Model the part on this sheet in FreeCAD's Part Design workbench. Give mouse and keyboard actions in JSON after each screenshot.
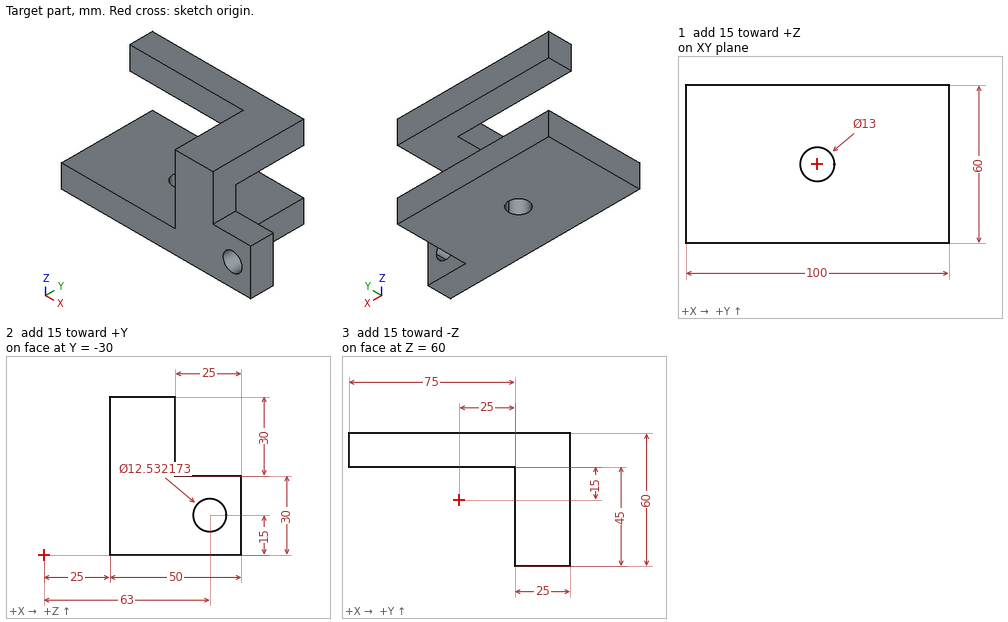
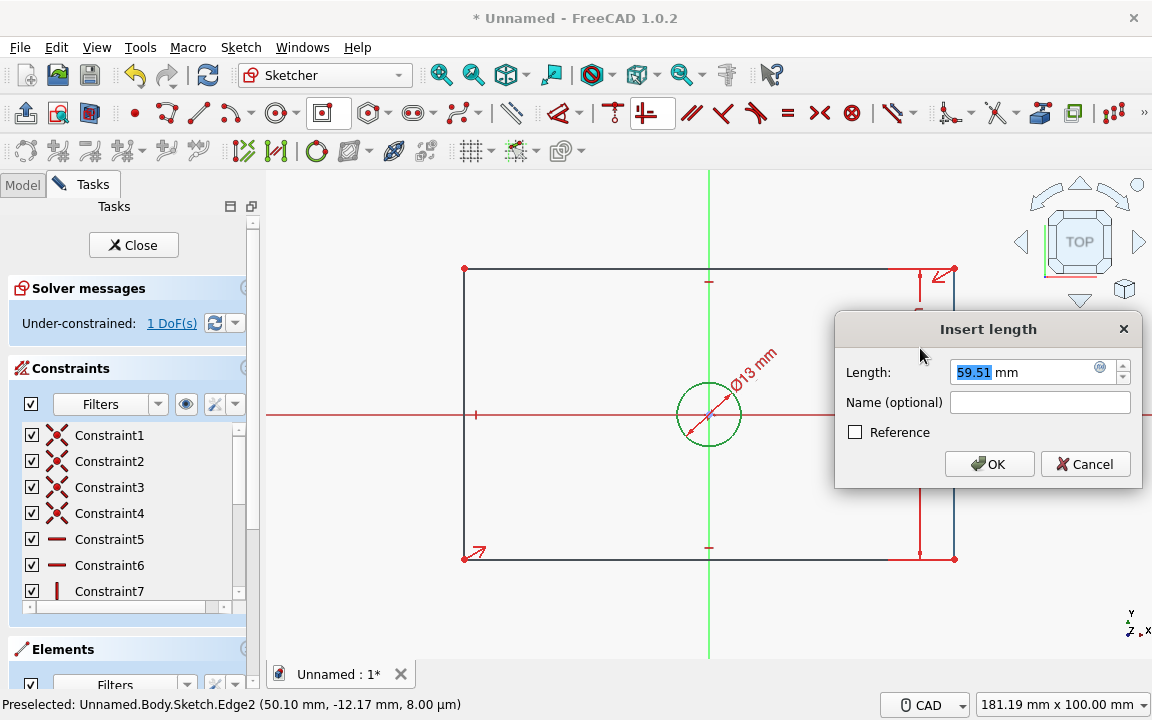
{"action": "type", "text": "60"}
{"action": "key", "text": "Return"}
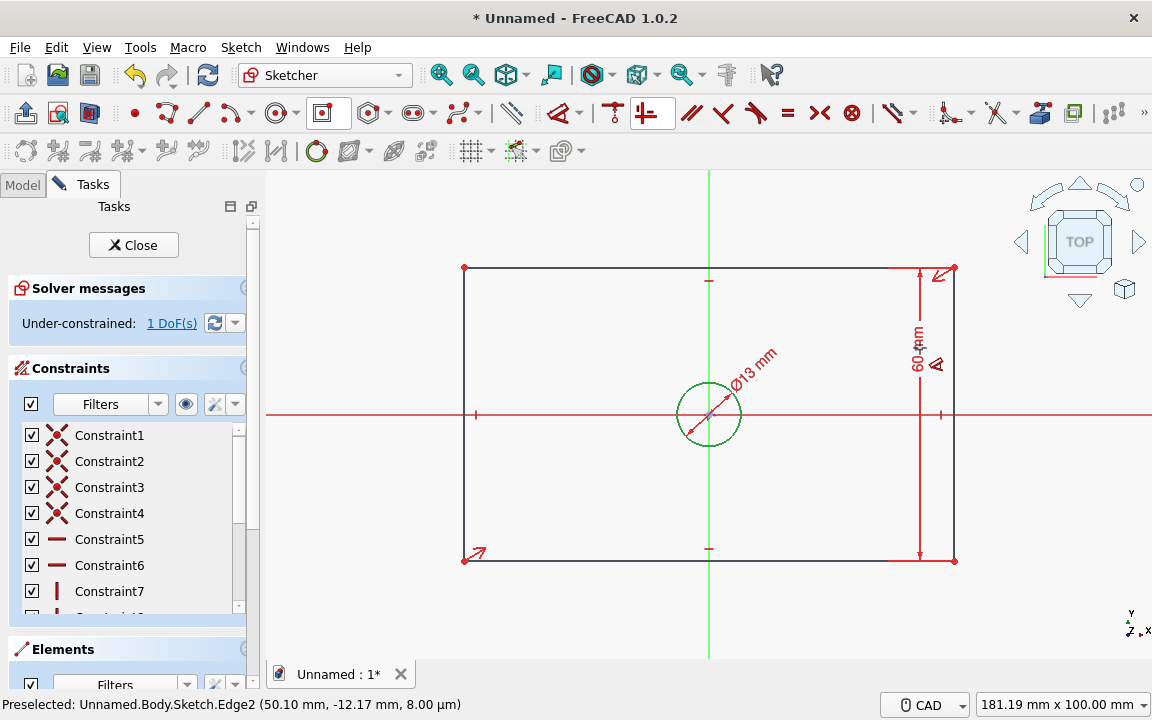
{"action": "left_click", "coordinate": [611, 561]}
{"action": "left_click", "coordinate": [596, 595]}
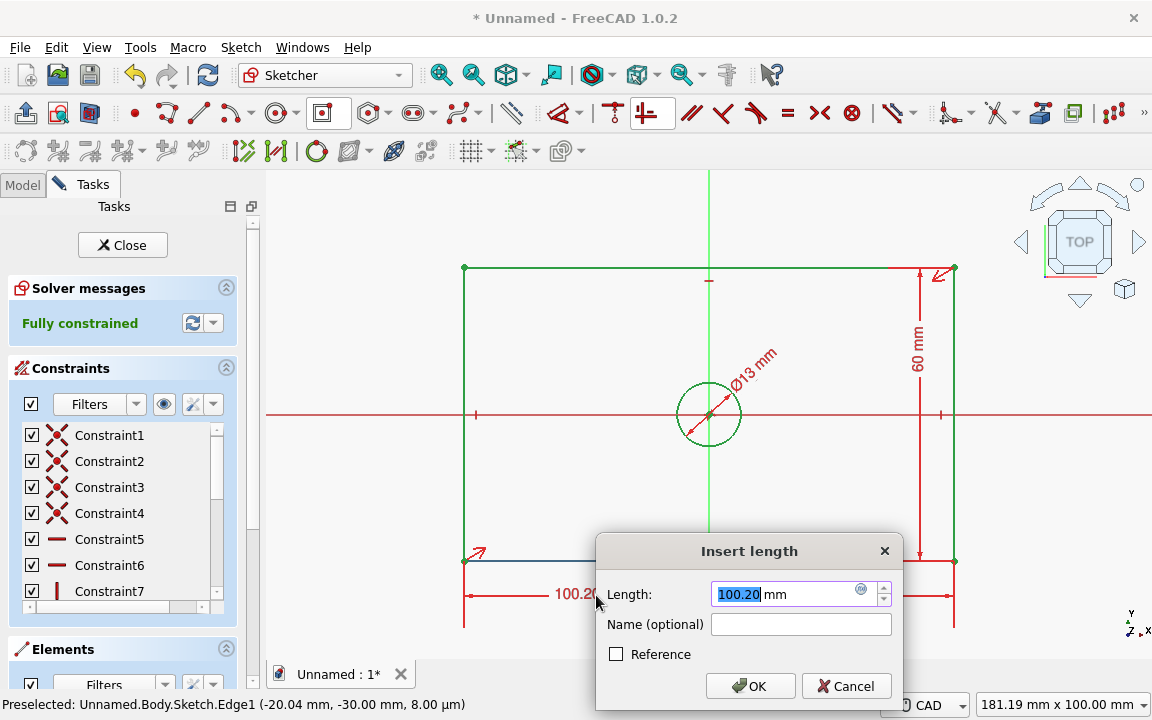
{"action": "type", "text": "100"}
{"action": "key", "text": "Return"}
{"action": "key", "text": "Escape"}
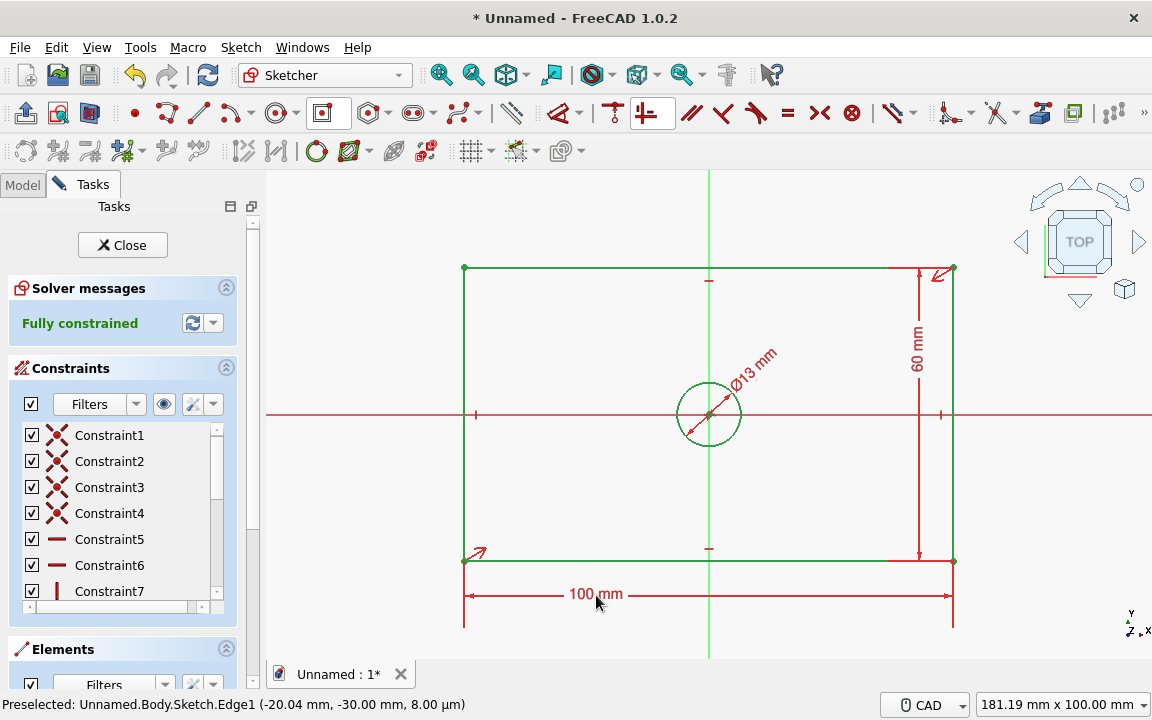
{"action": "left_click", "coordinate": [123, 245]}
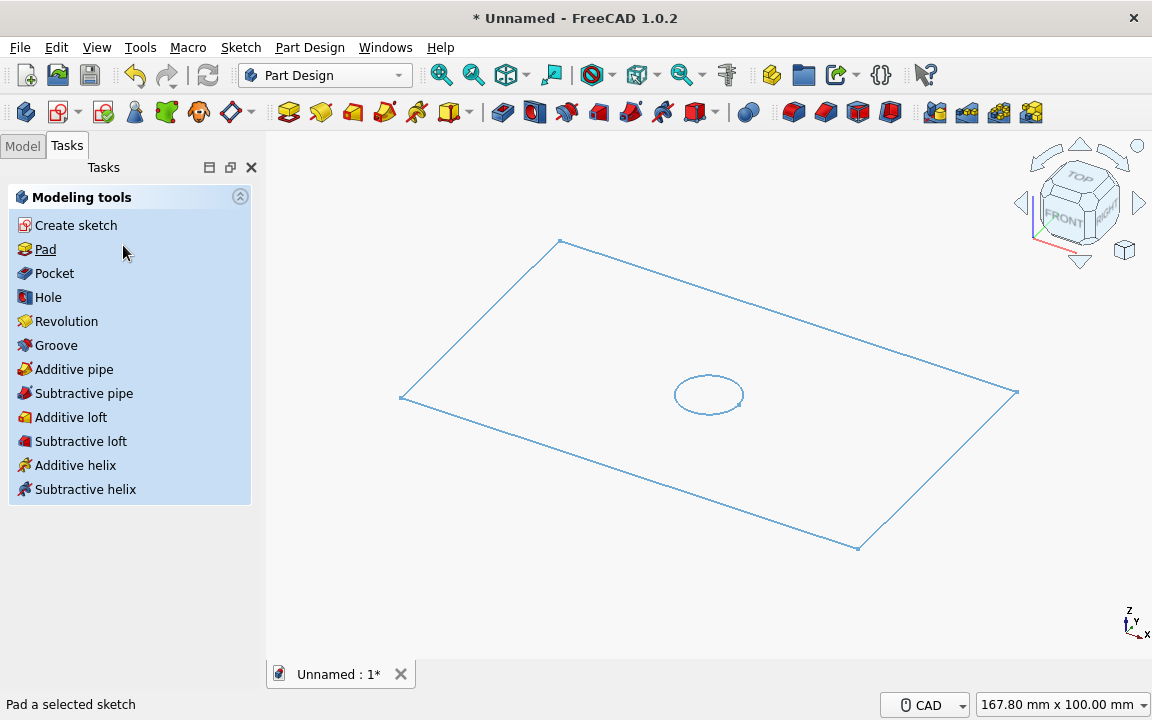
{"action": "left_click", "coordinate": [290, 112]}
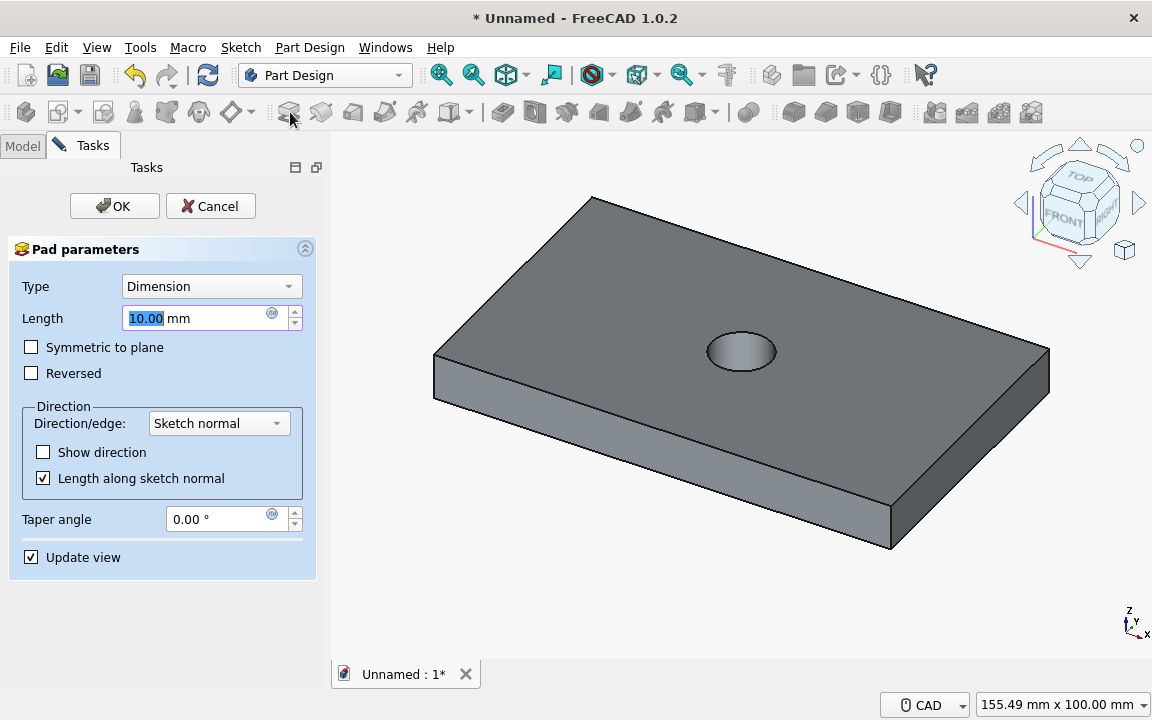
{"action": "type", "text": "15"}
{"action": "key", "text": "Tab"}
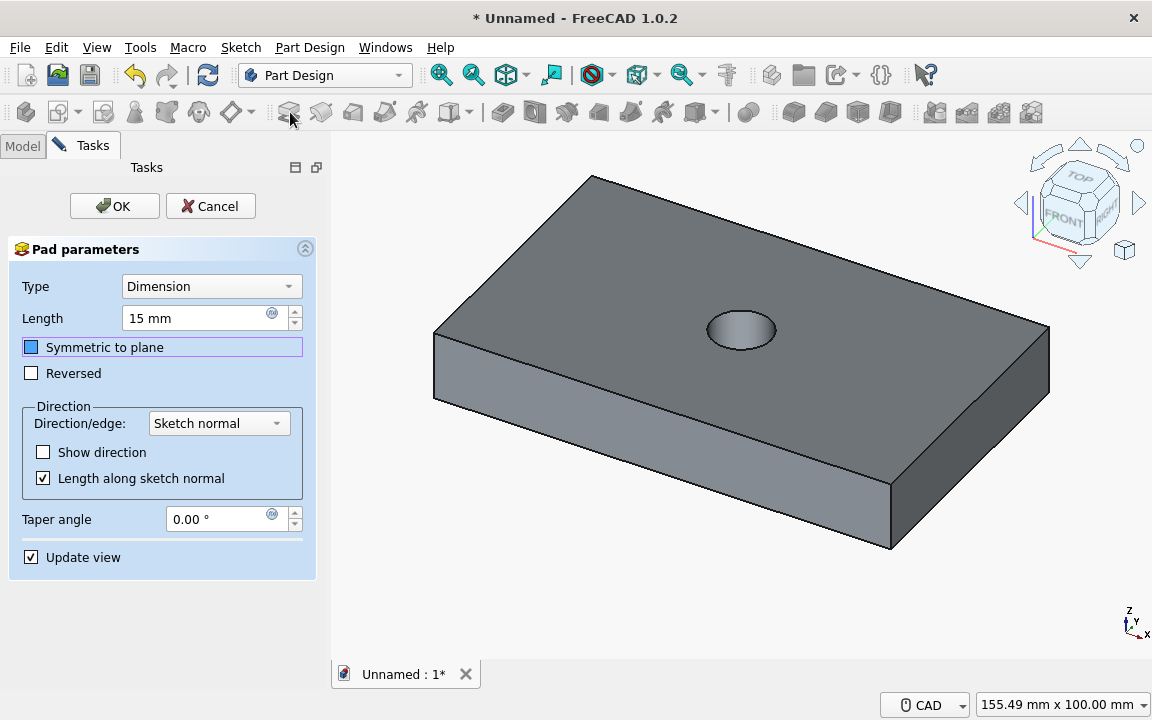
{"action": "left_click", "coordinate": [115, 206]}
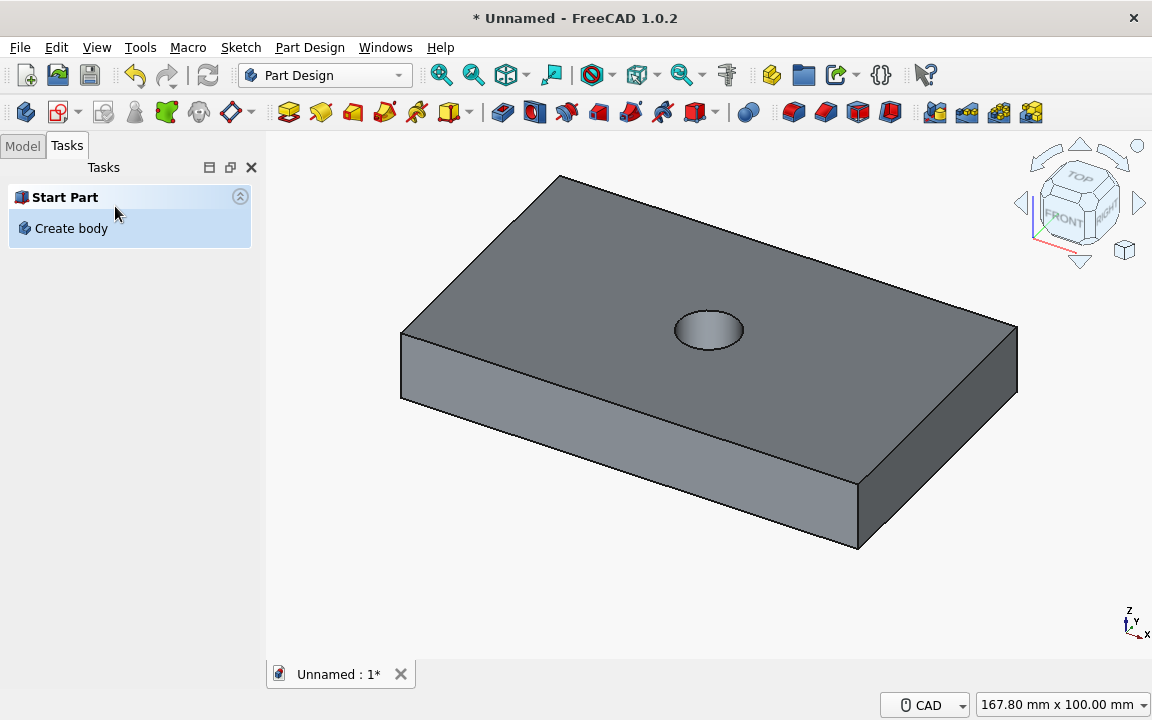
{"action": "left_click", "coordinate": [760, 484]}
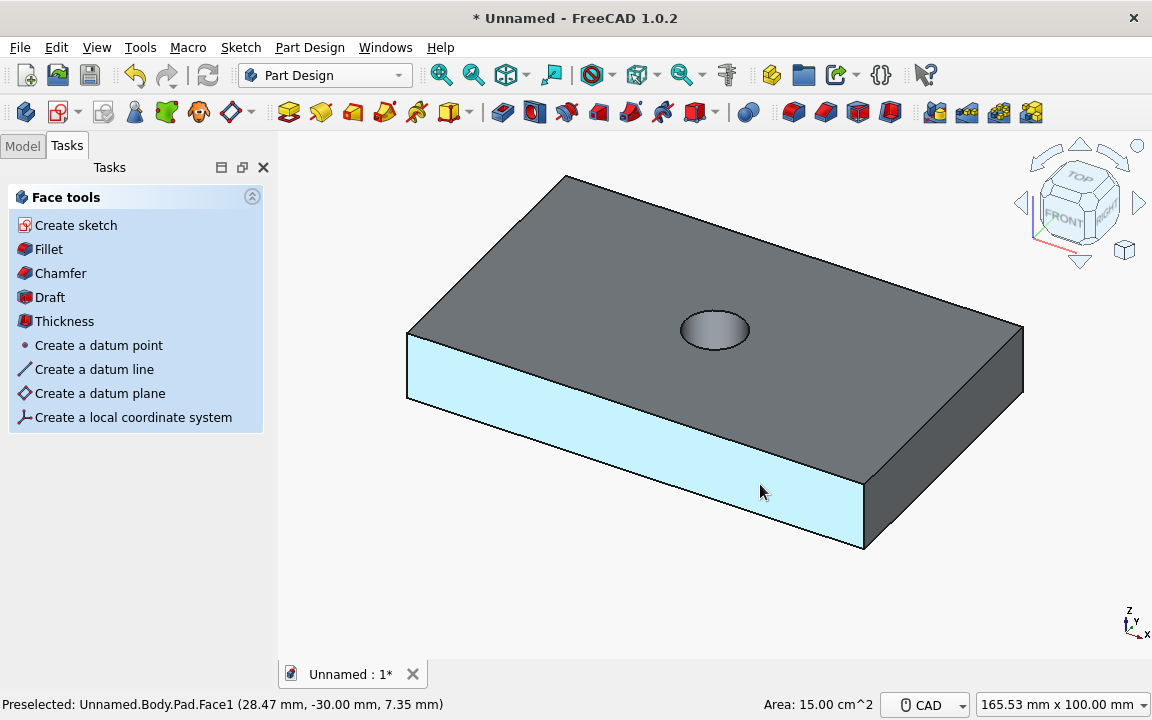
{"action": "left_click", "coordinate": [58, 112]}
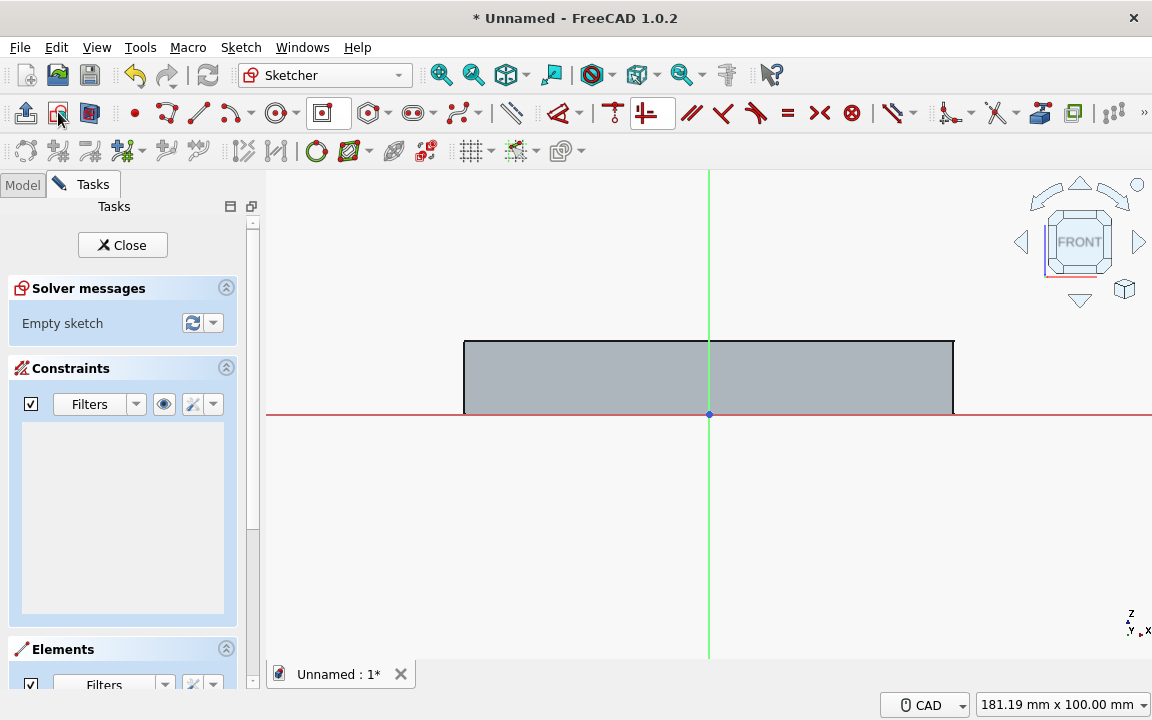
{"action": "scroll", "coordinate": [294, 631], "scroll_direction": "down", "scroll_amount": 2}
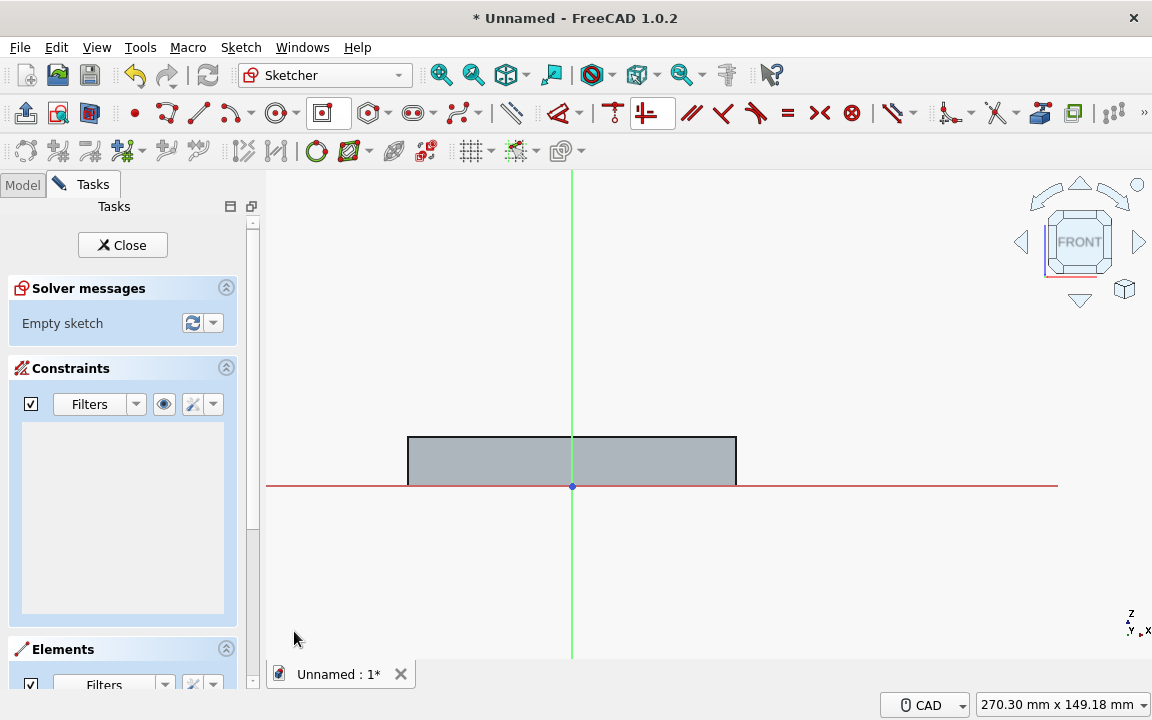
{"action": "scroll", "coordinate": [806, 334], "scroll_direction": "up", "scroll_amount": 2}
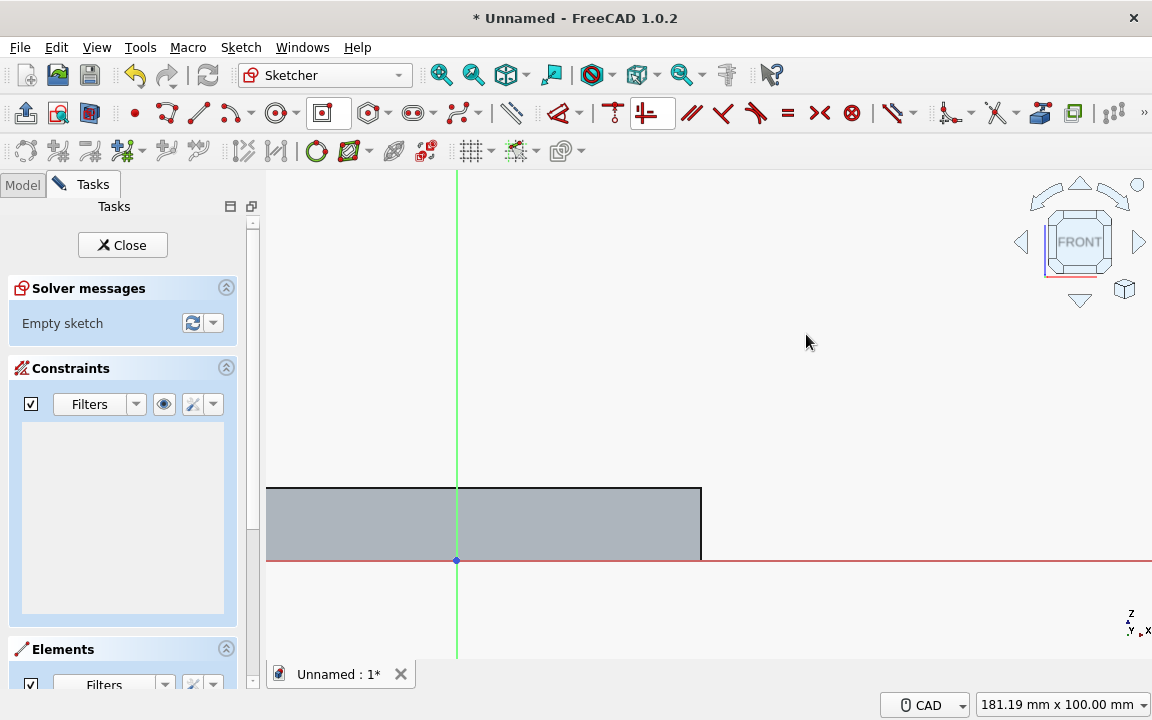
{"action": "key", "text": "g m"}